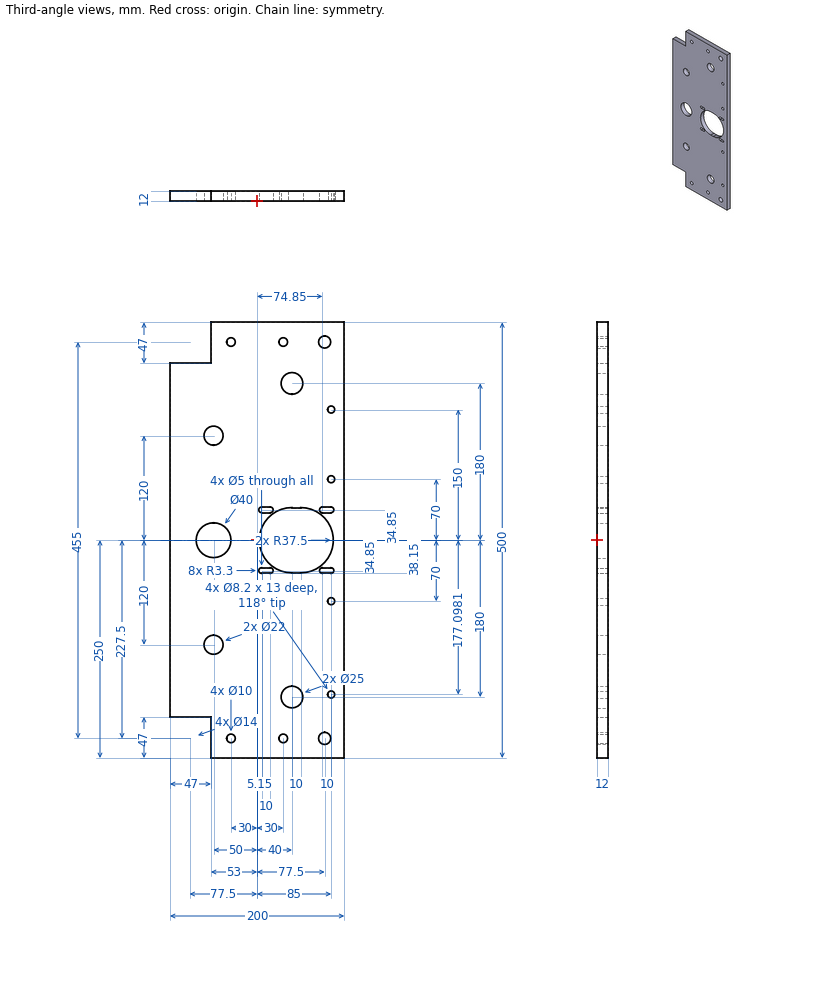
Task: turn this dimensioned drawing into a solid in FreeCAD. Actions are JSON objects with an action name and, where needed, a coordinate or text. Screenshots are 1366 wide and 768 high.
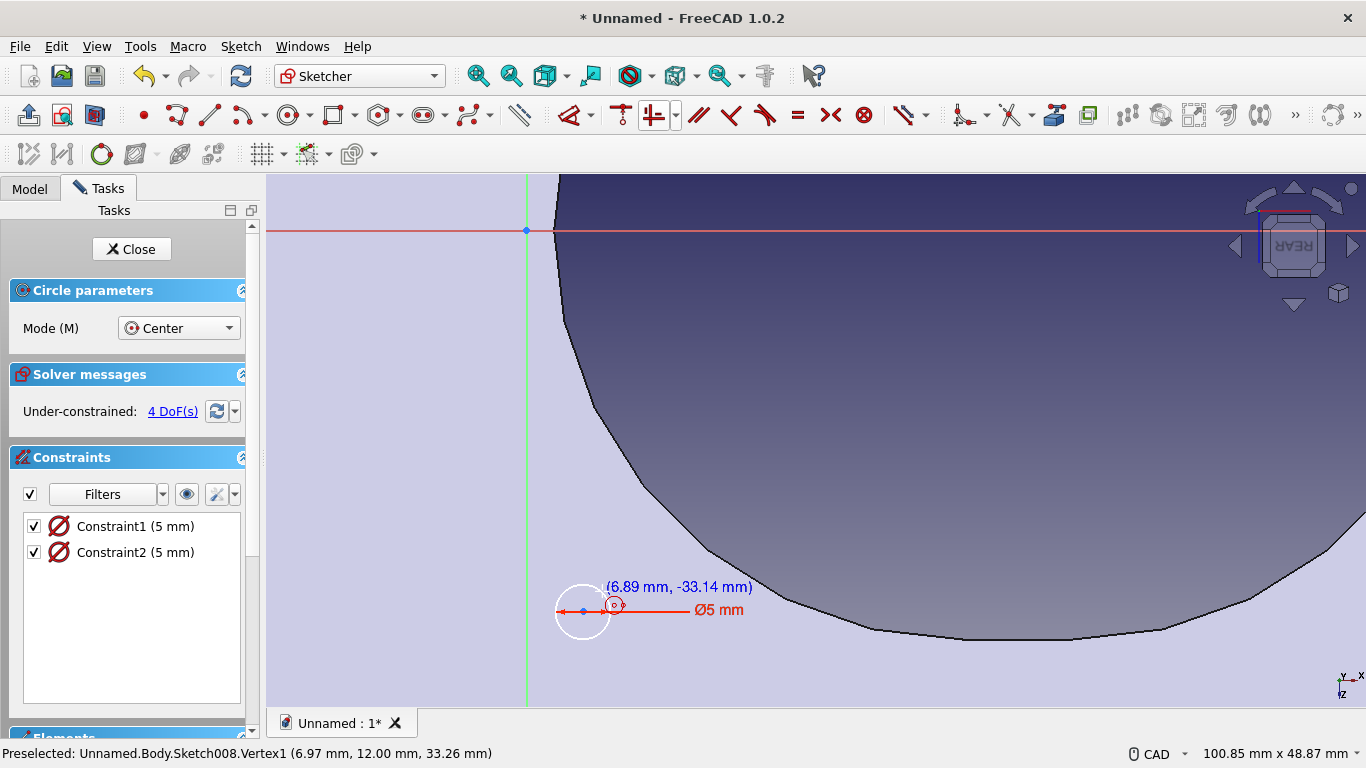
{"action": "scroll", "coordinate": [583, 612], "scroll_direction": "down", "scroll_amount": 4}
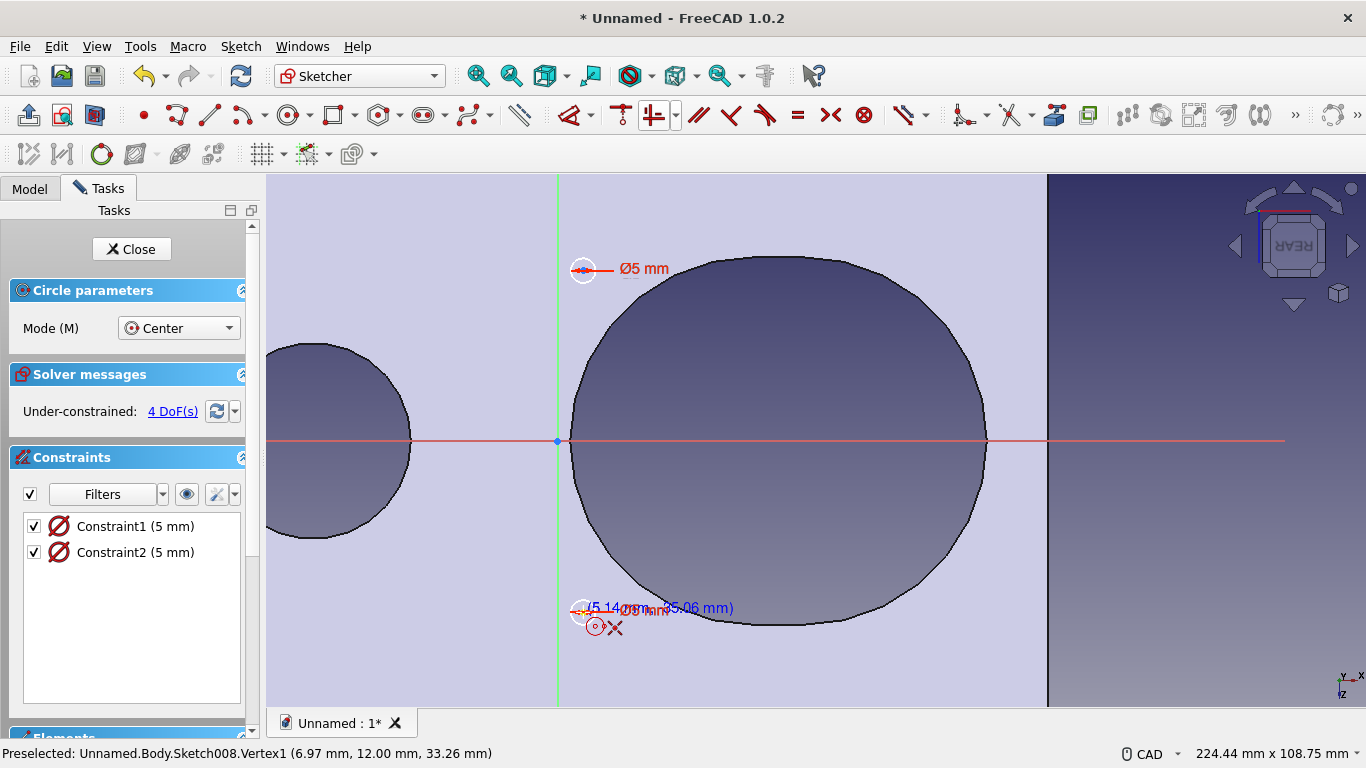
{"action": "scroll", "coordinate": [925, 612], "scroll_direction": "up", "scroll_amount": 4}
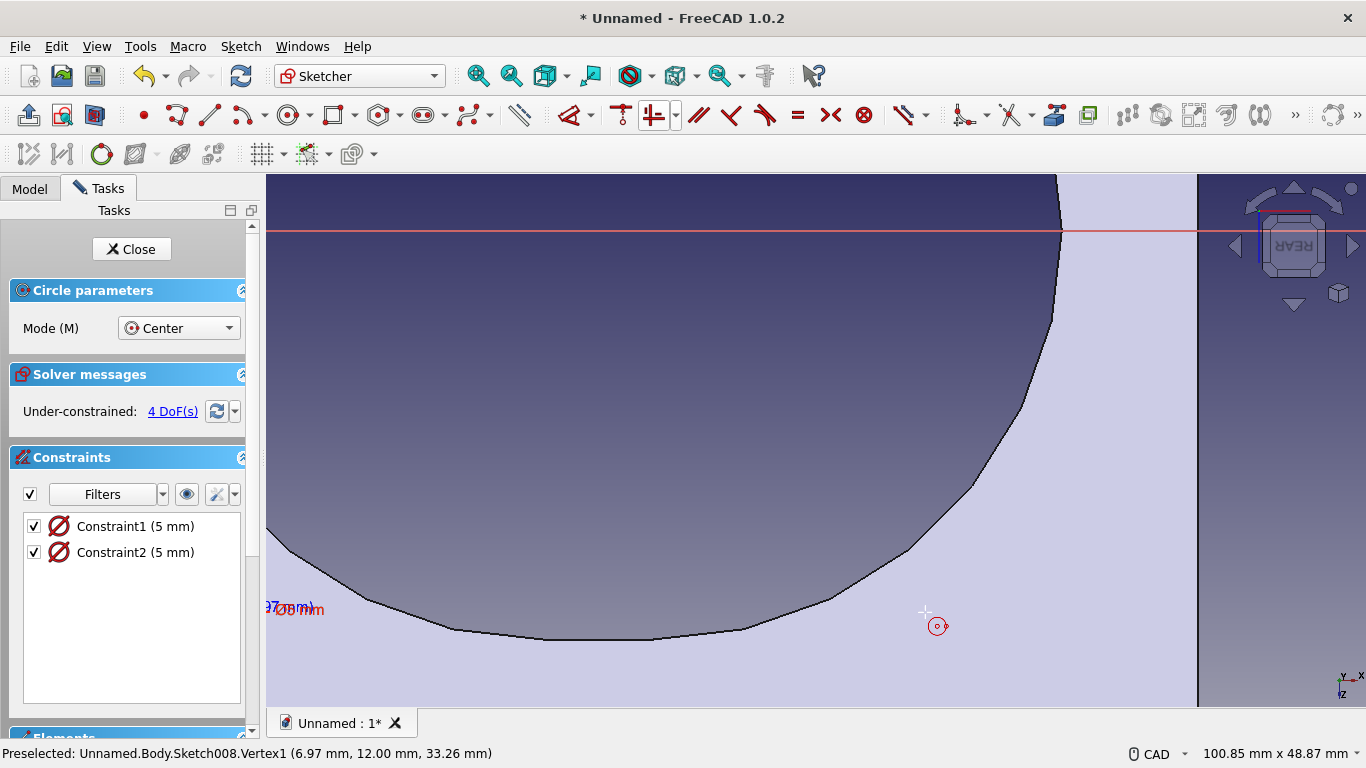
{"action": "left_click", "coordinate": [924, 611]}
{"action": "mouse_move", "coordinate": [943, 591]}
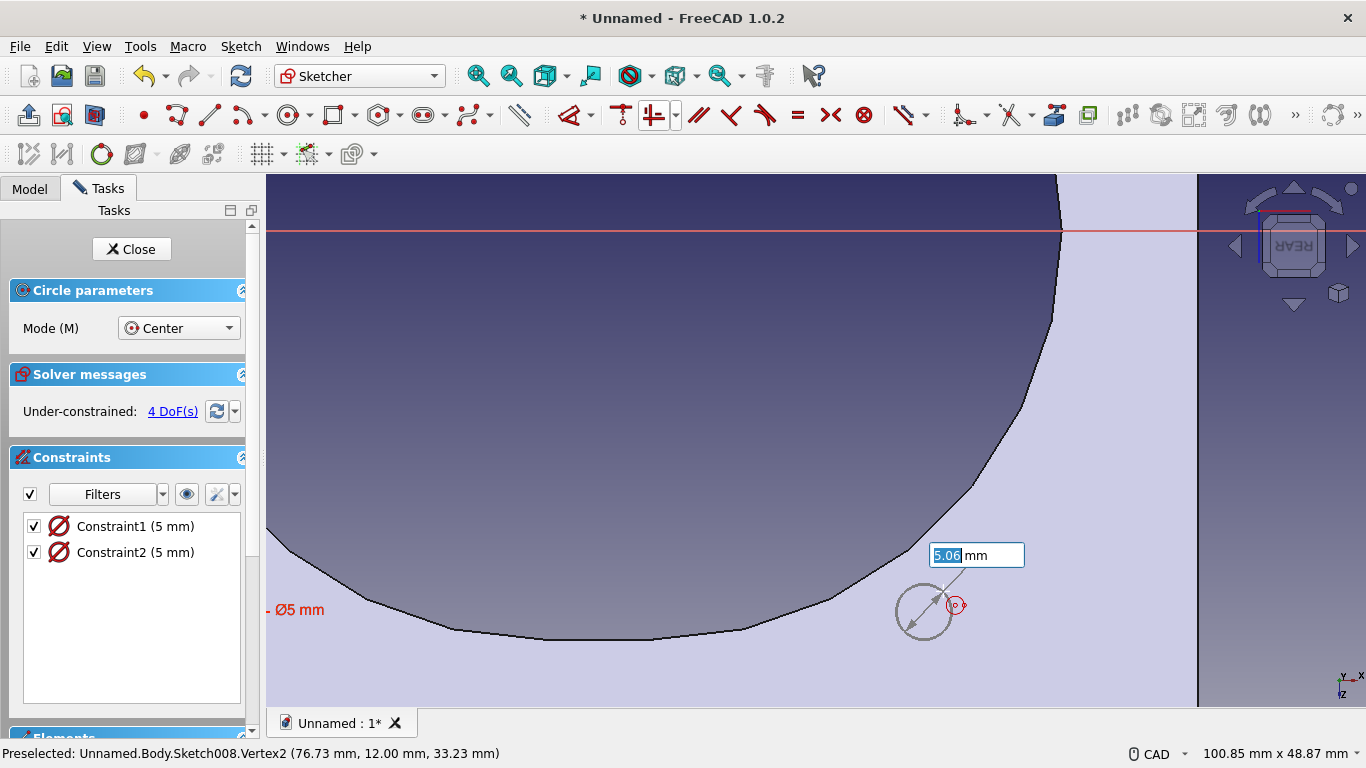
{"action": "type", "text": "5"}
{"action": "key", "text": "Return"}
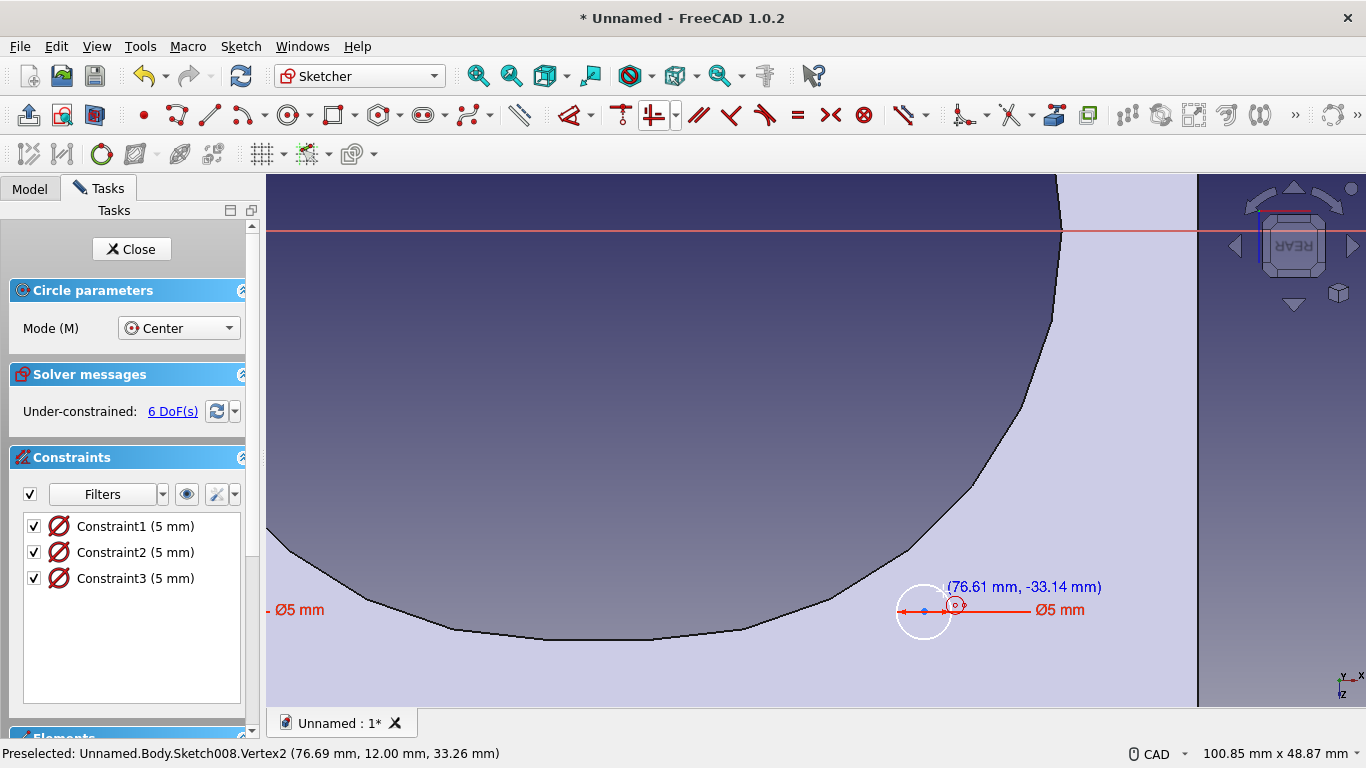
{"action": "scroll", "coordinate": [926, 612], "scroll_direction": "down", "scroll_amount": 4}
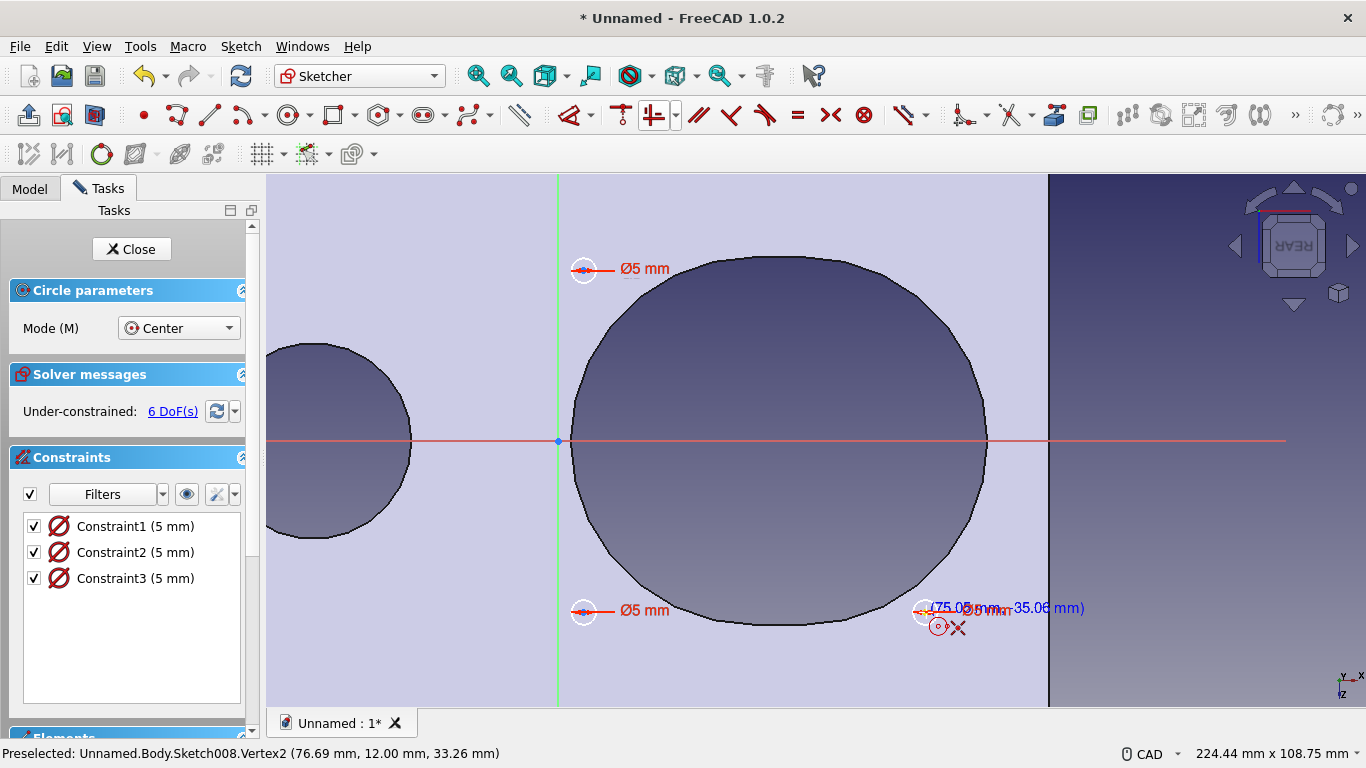
{"action": "scroll", "coordinate": [925, 270], "scroll_direction": "up", "scroll_amount": 4}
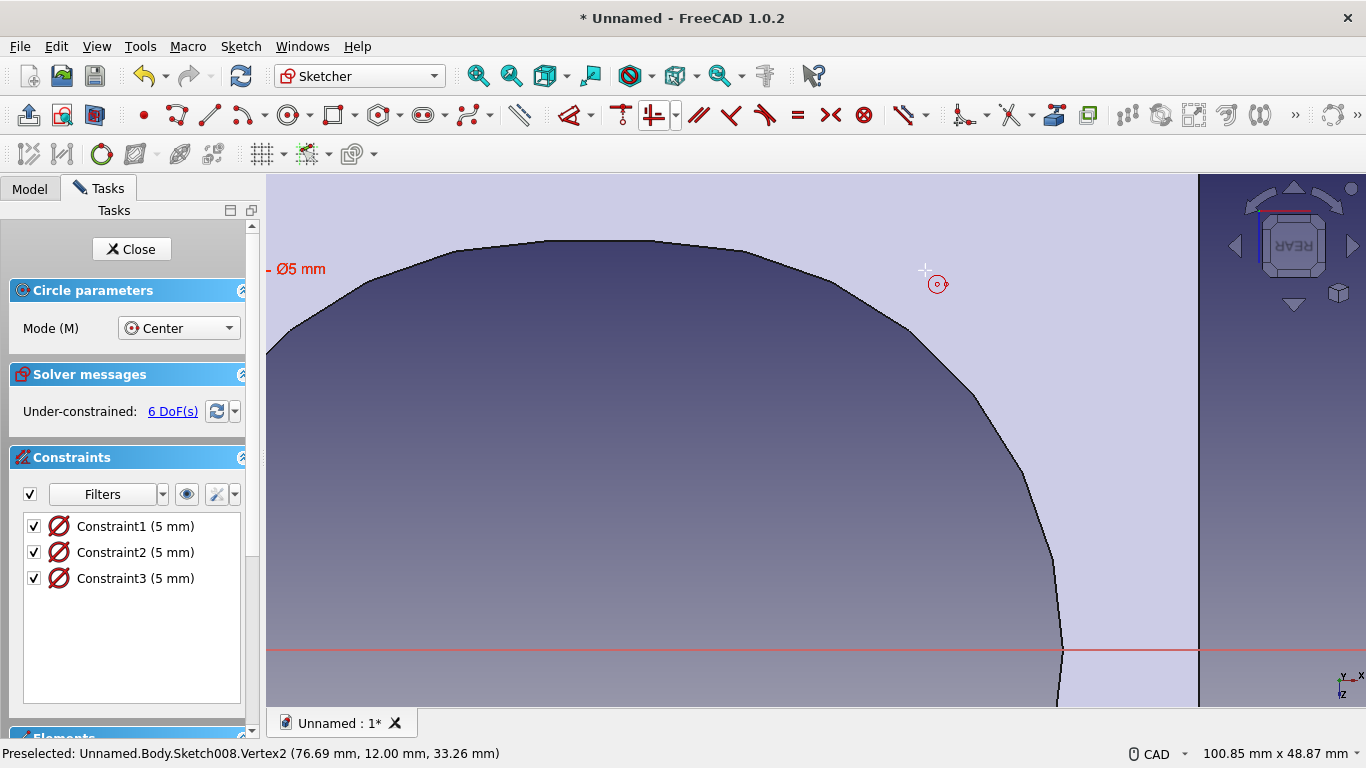
{"action": "left_click", "coordinate": [925, 270]}
{"action": "mouse_move", "coordinate": [944, 251]}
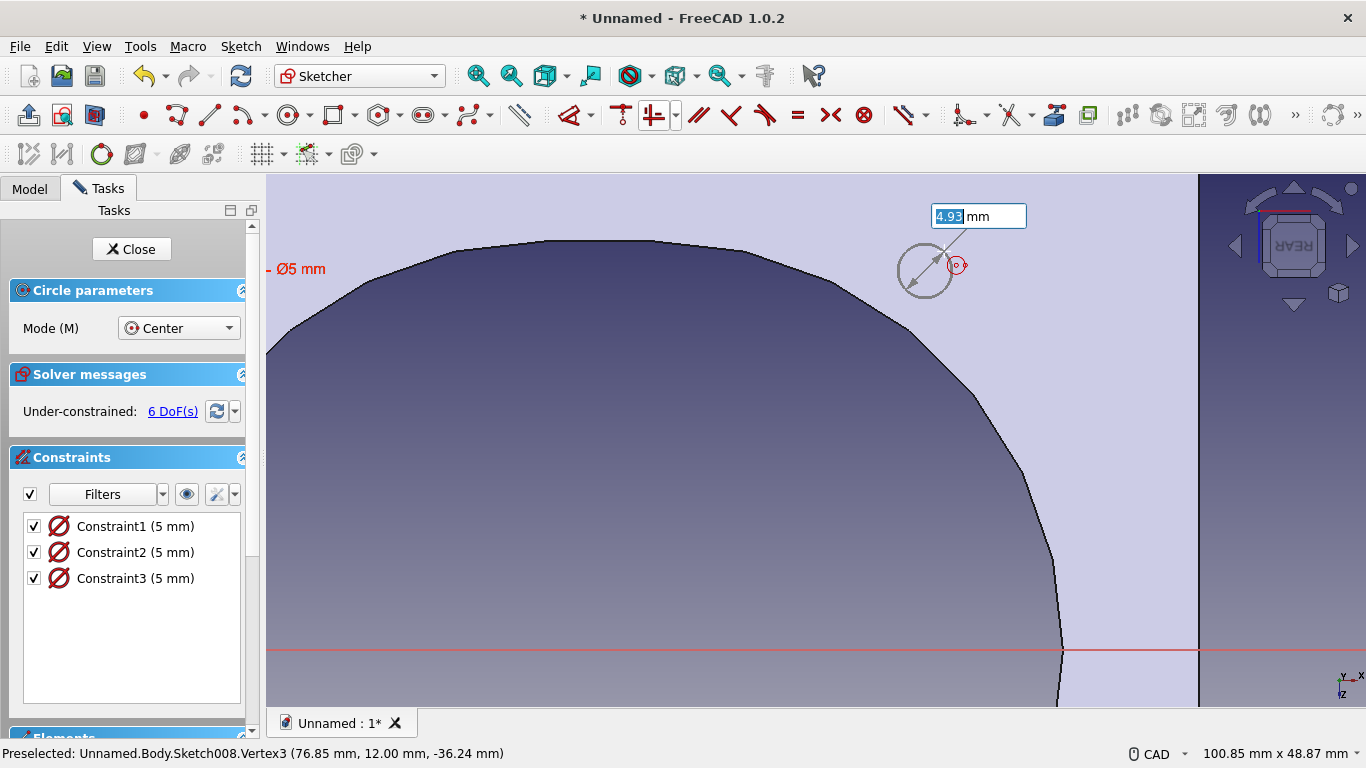
{"action": "type", "text": "5"}
{"action": "key", "text": "Return"}
{"action": "key", "text": "Escape"}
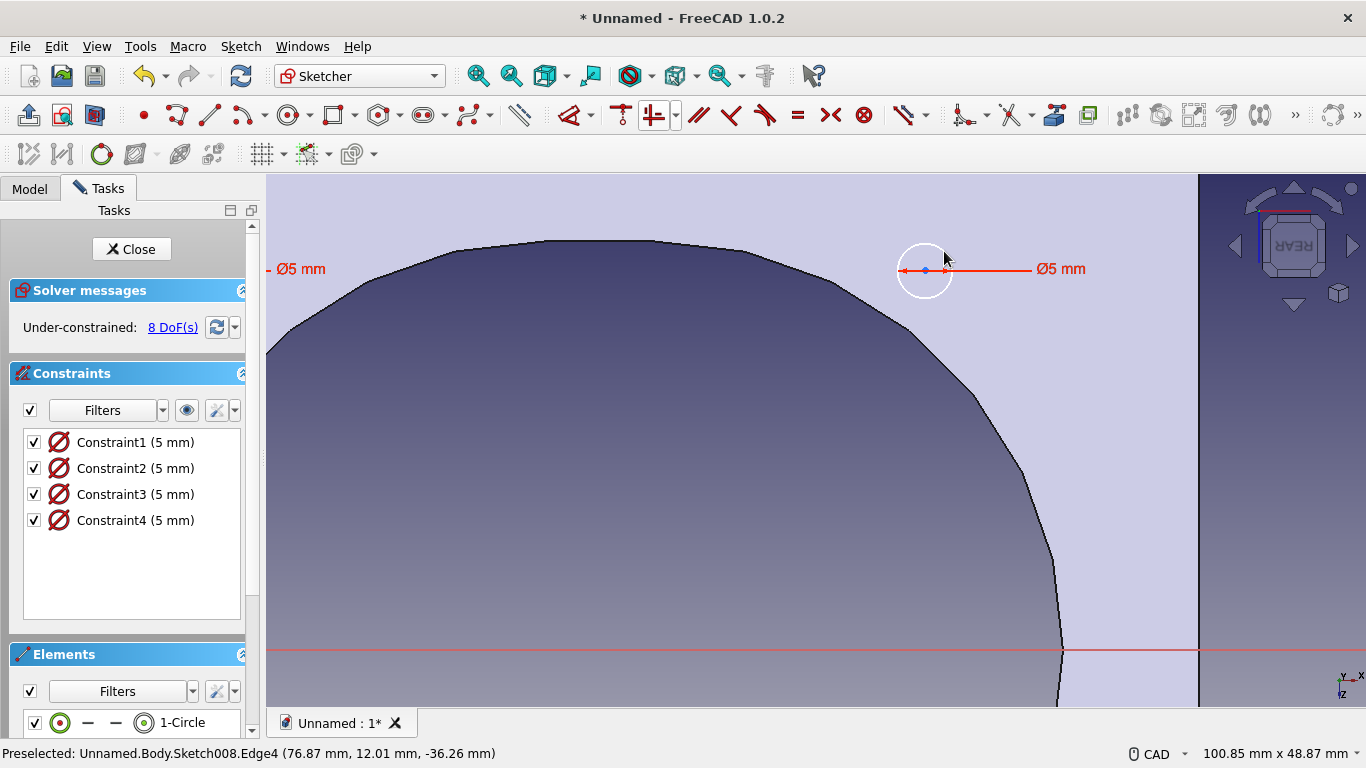
{"action": "scroll", "coordinate": [925, 269], "scroll_direction": "down", "scroll_amount": 4}